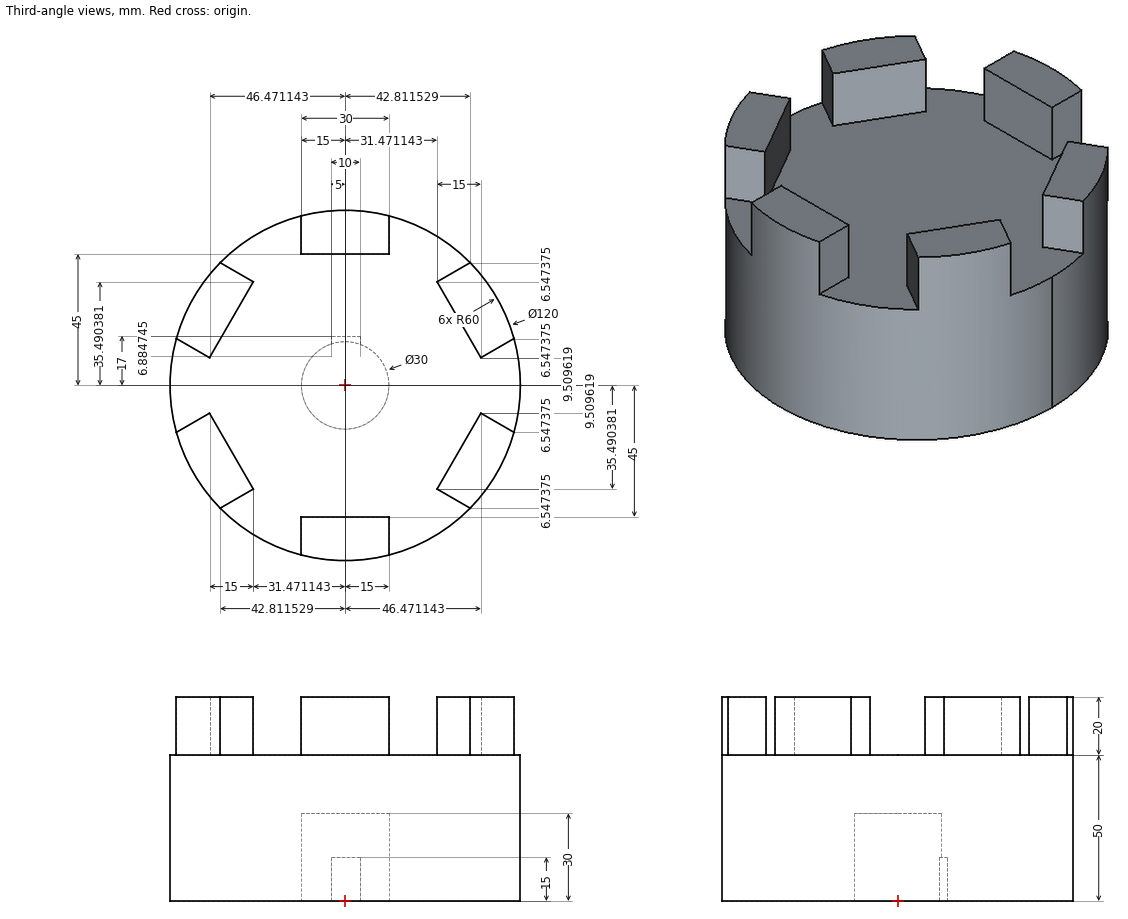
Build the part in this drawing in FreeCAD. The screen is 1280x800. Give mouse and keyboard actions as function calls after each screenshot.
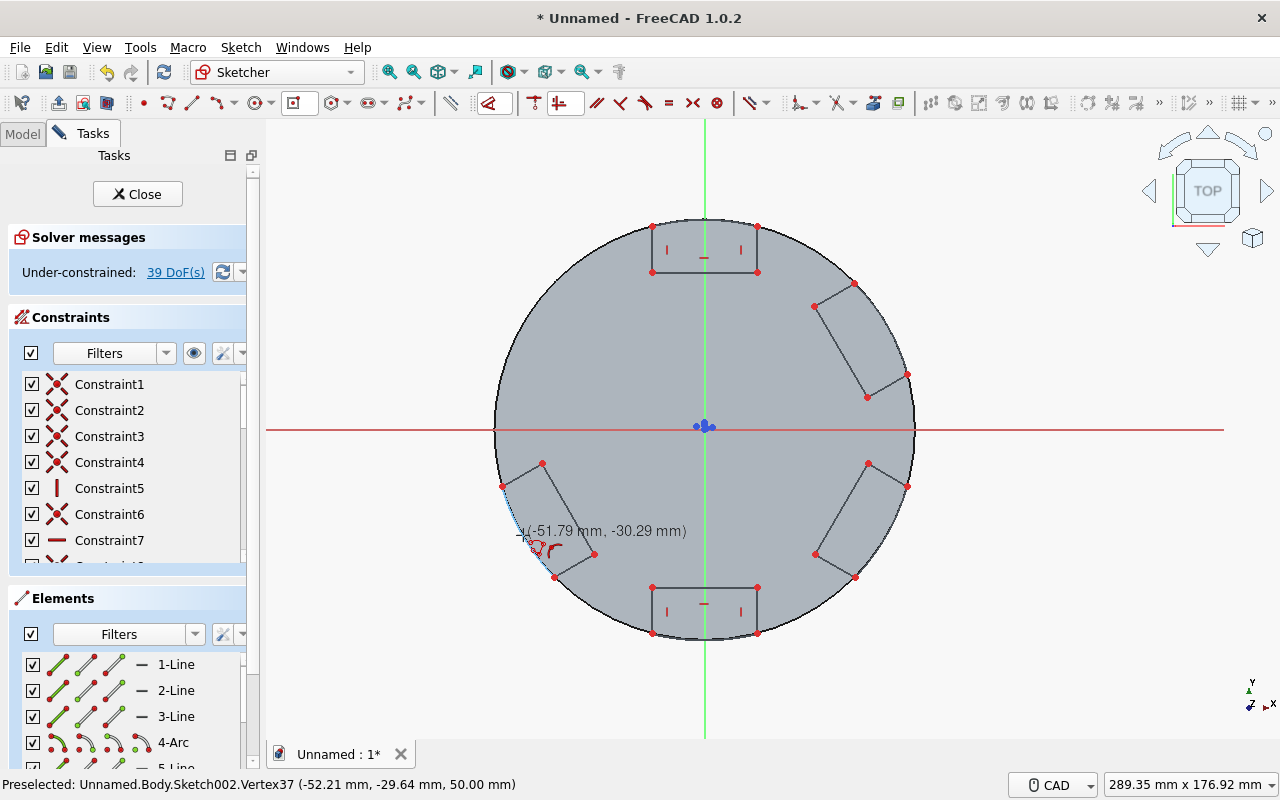
click(502, 373)
click(542, 396)
click(594, 305)
click(555, 282)
right_click(555, 282)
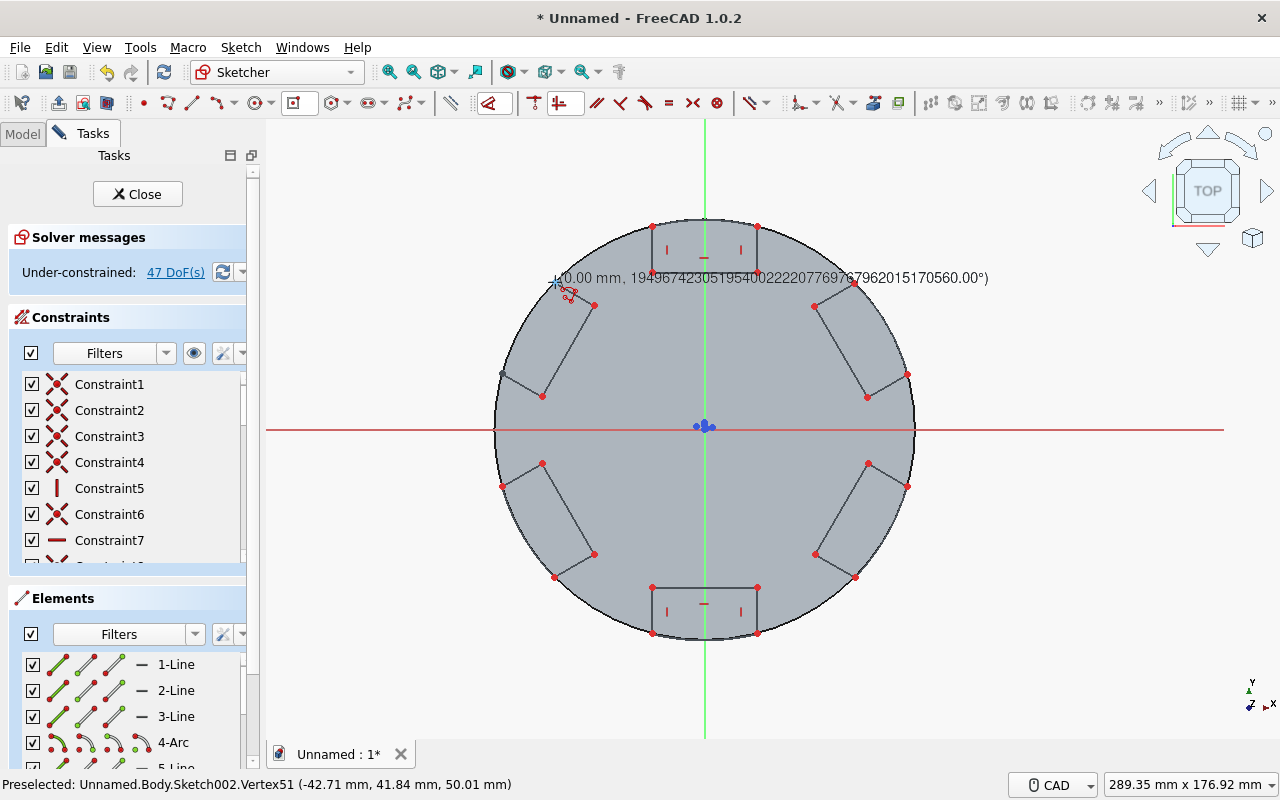
click(218, 104)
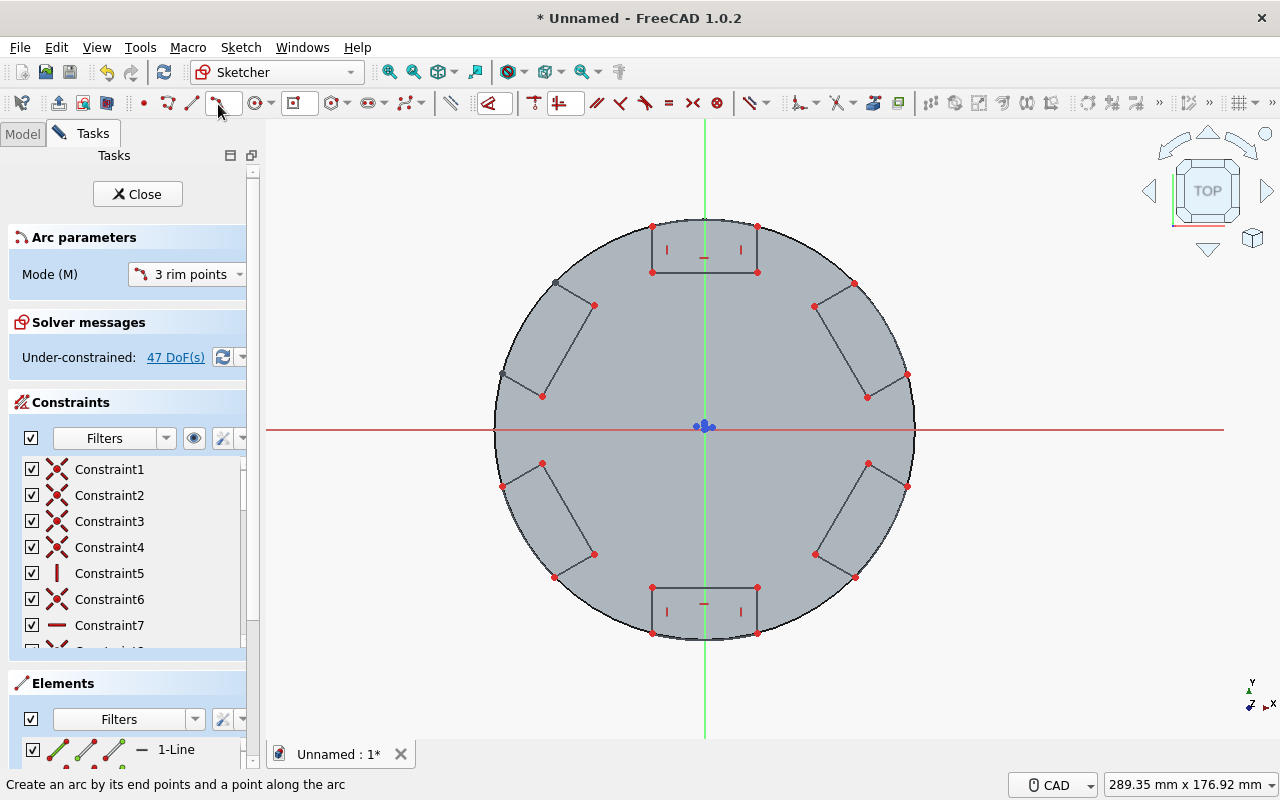
click(555, 283)
click(502, 374)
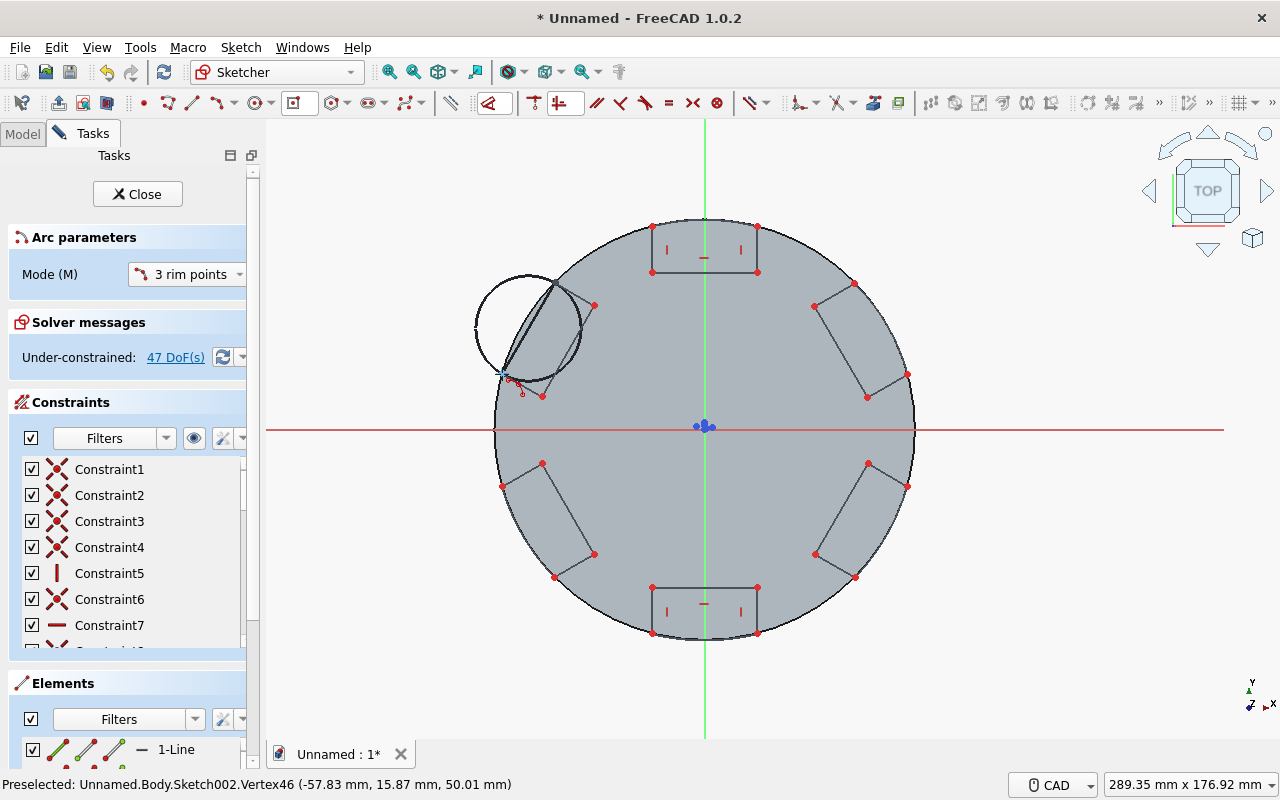
scroll(523, 324, up, 5)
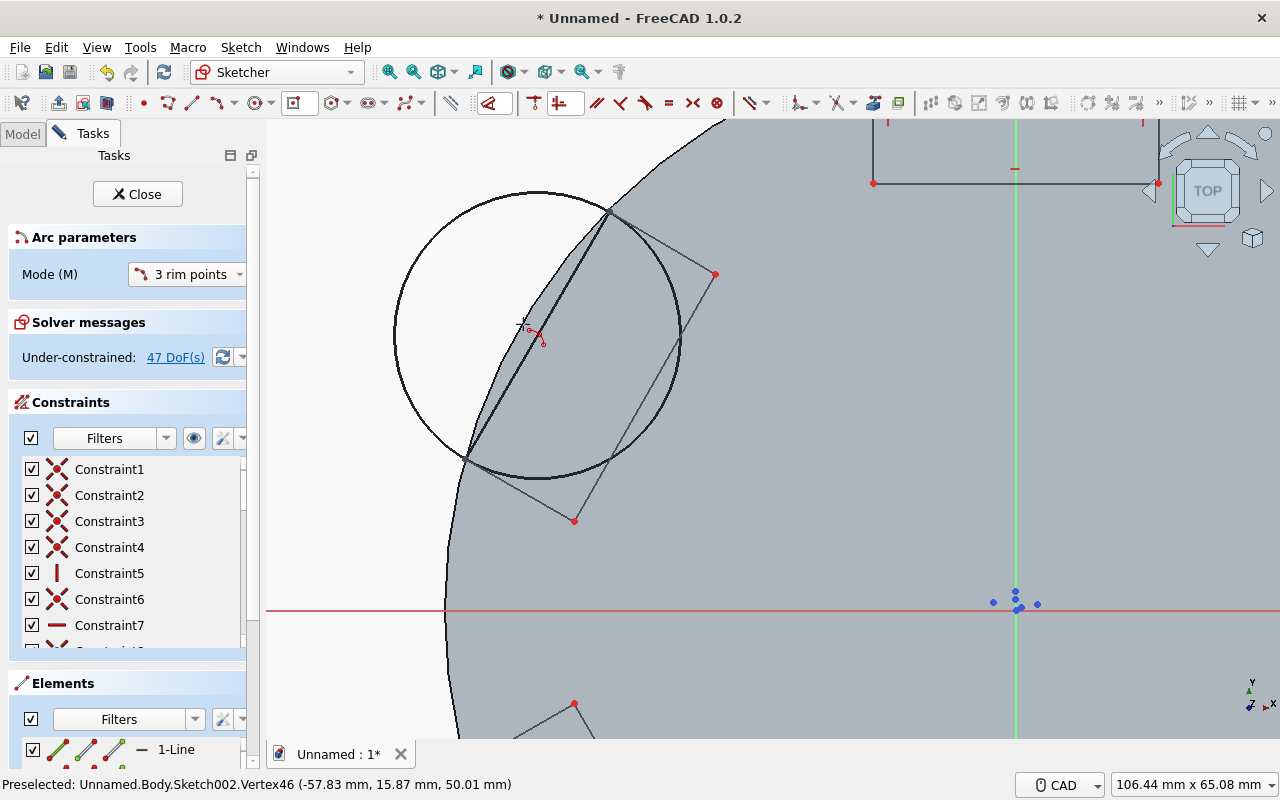
click(521, 325)
key(Escape)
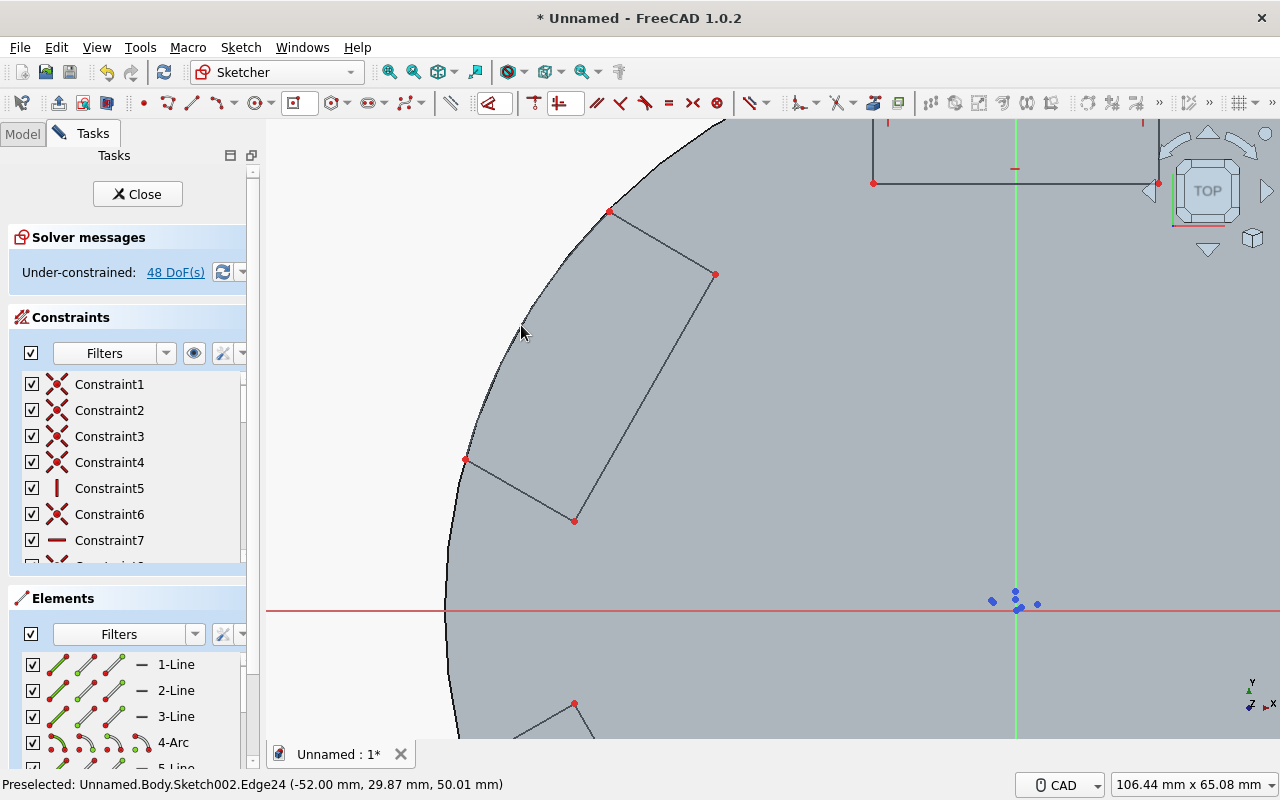
scroll(523, 323, down, 5)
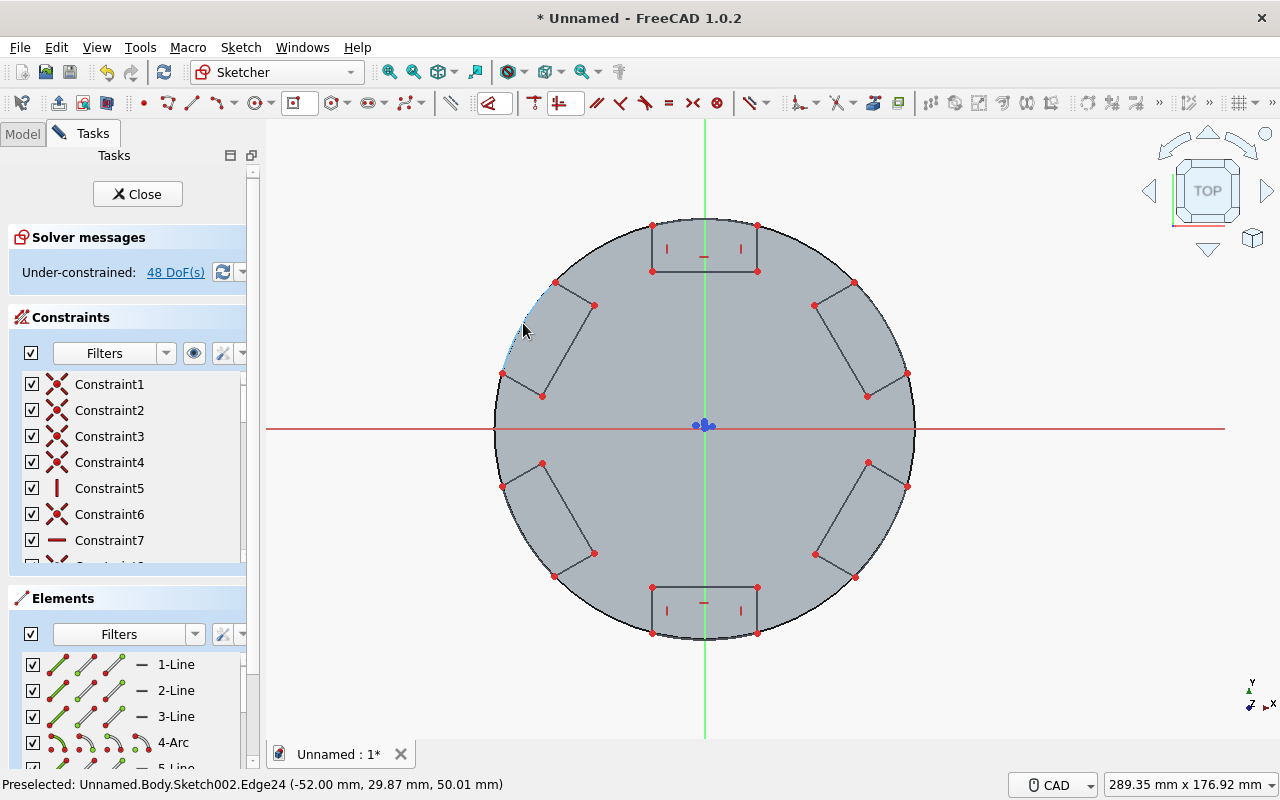
click(897, 344)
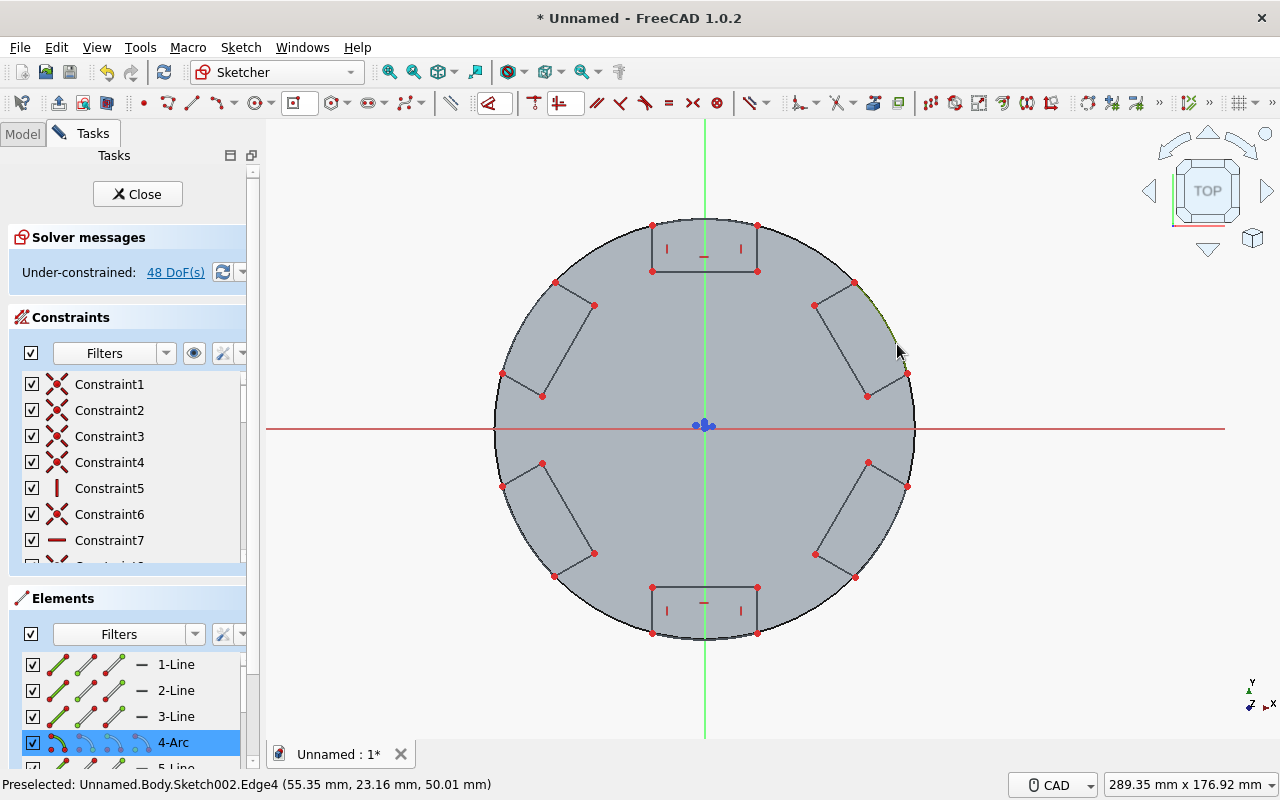
click(726, 220)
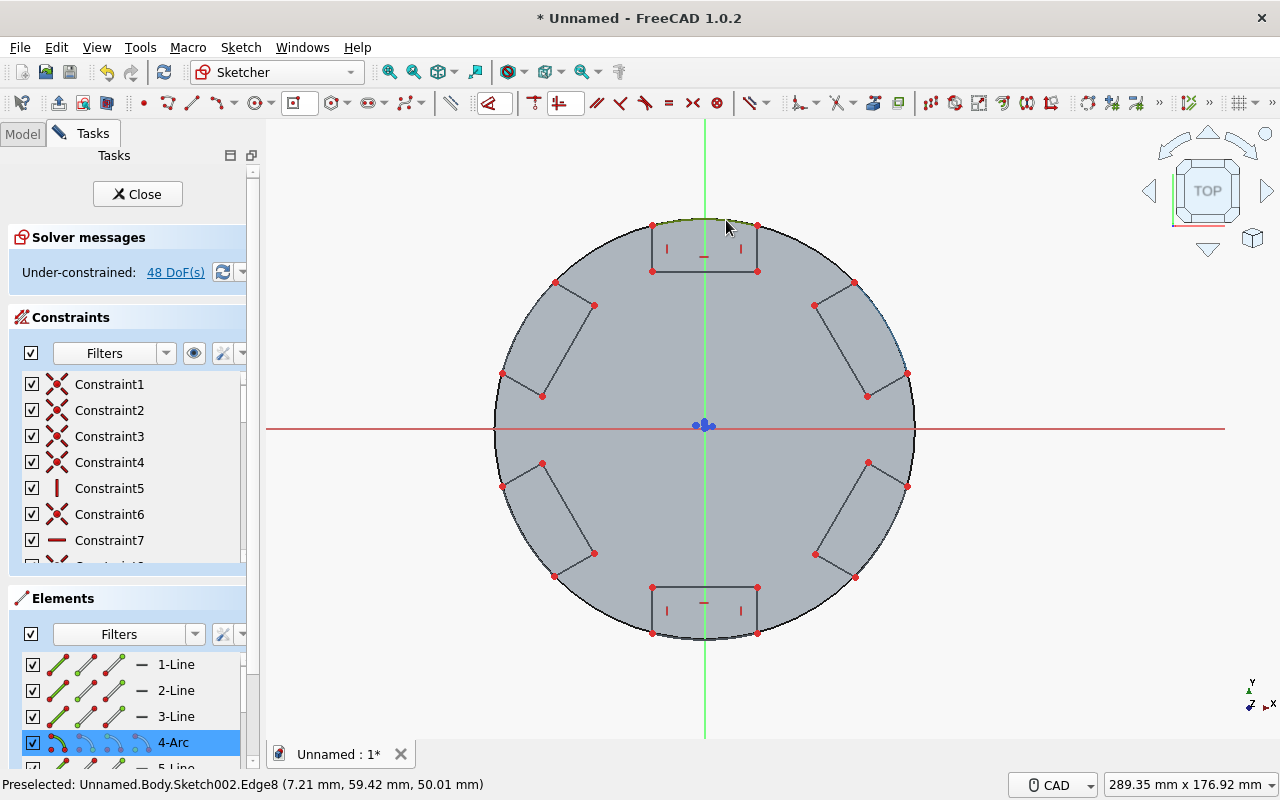
click(534, 104)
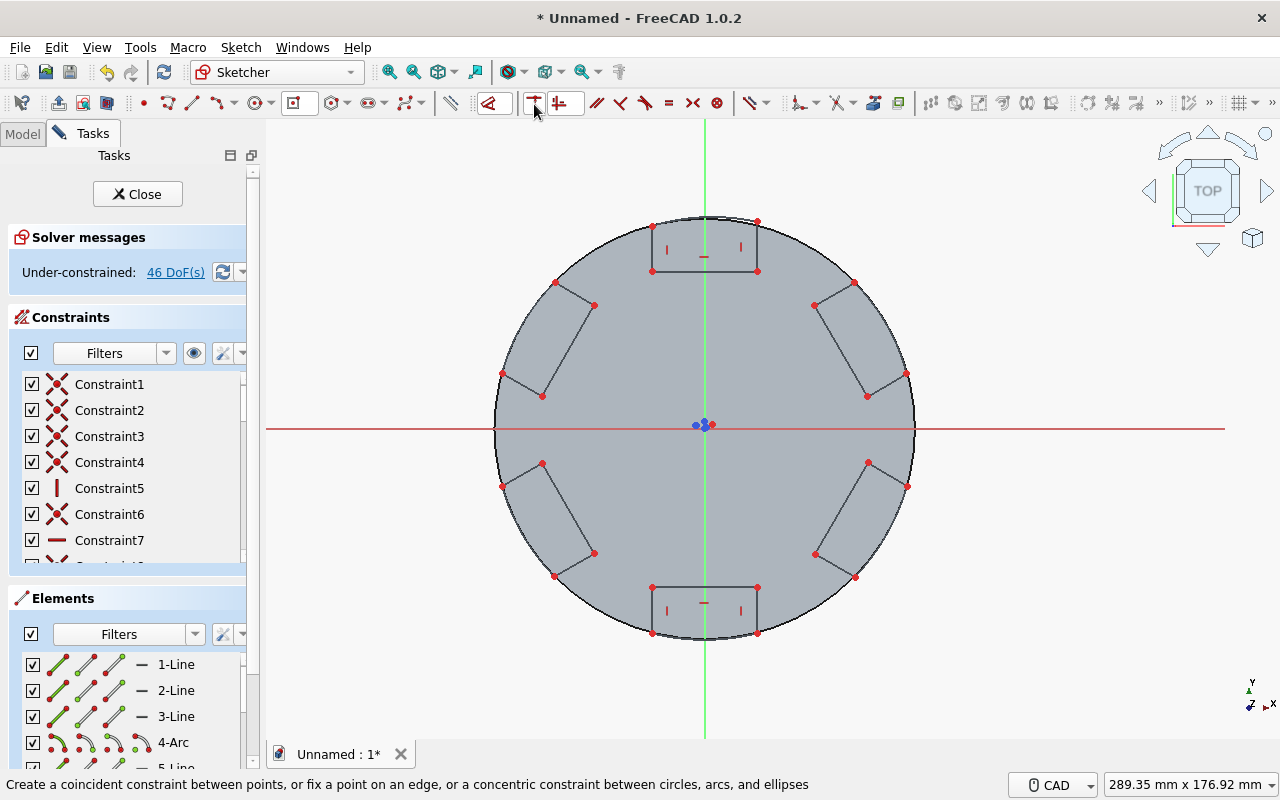
click(896, 344)